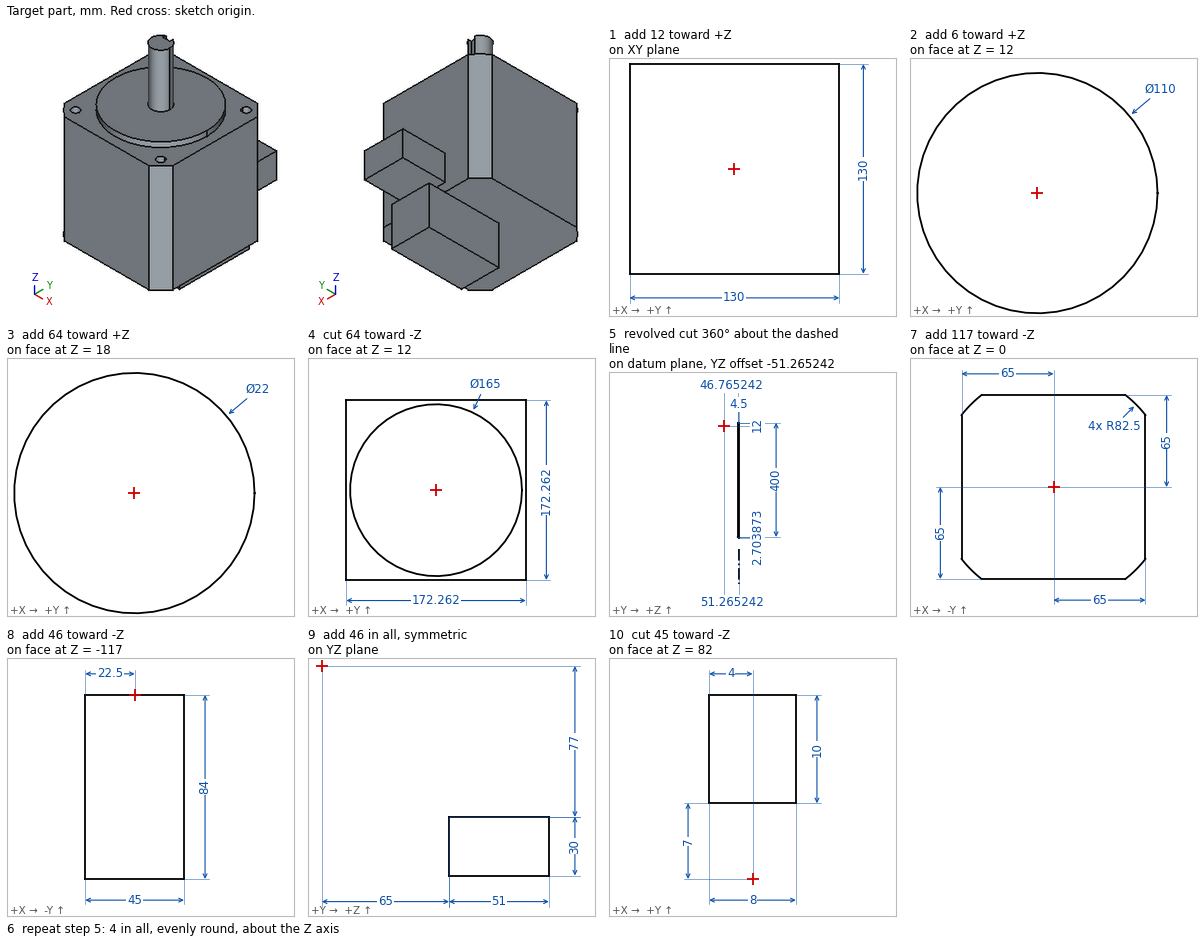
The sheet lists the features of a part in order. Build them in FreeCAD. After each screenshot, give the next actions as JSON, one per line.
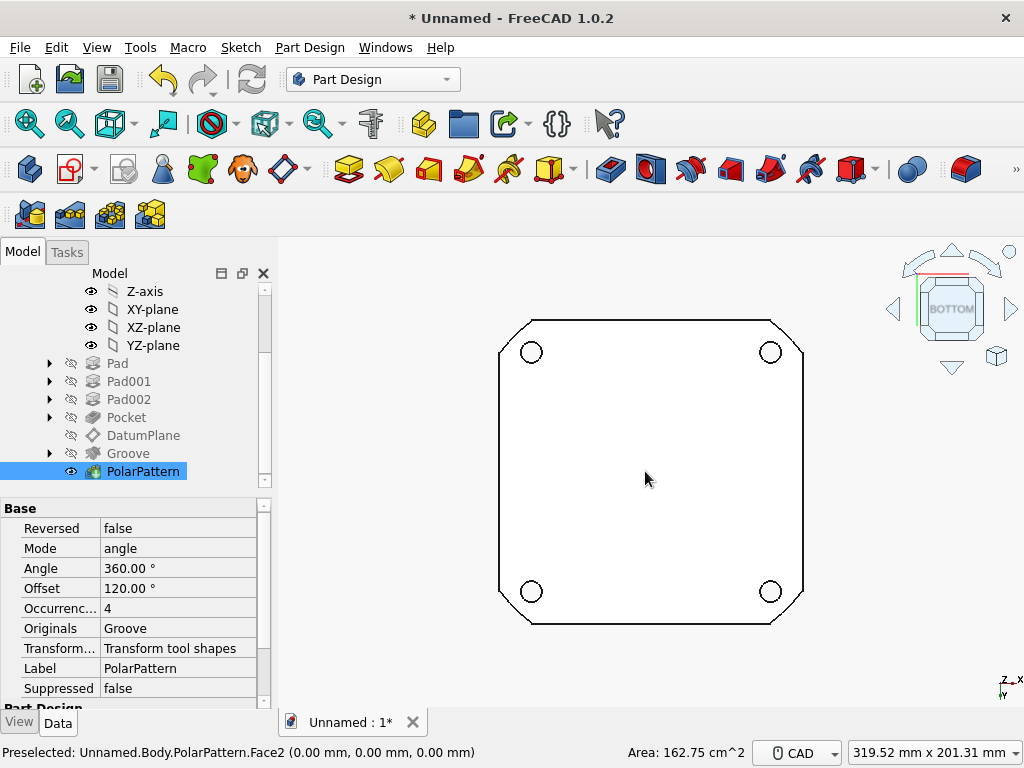
{"action": "left_click", "coordinate": [70, 170]}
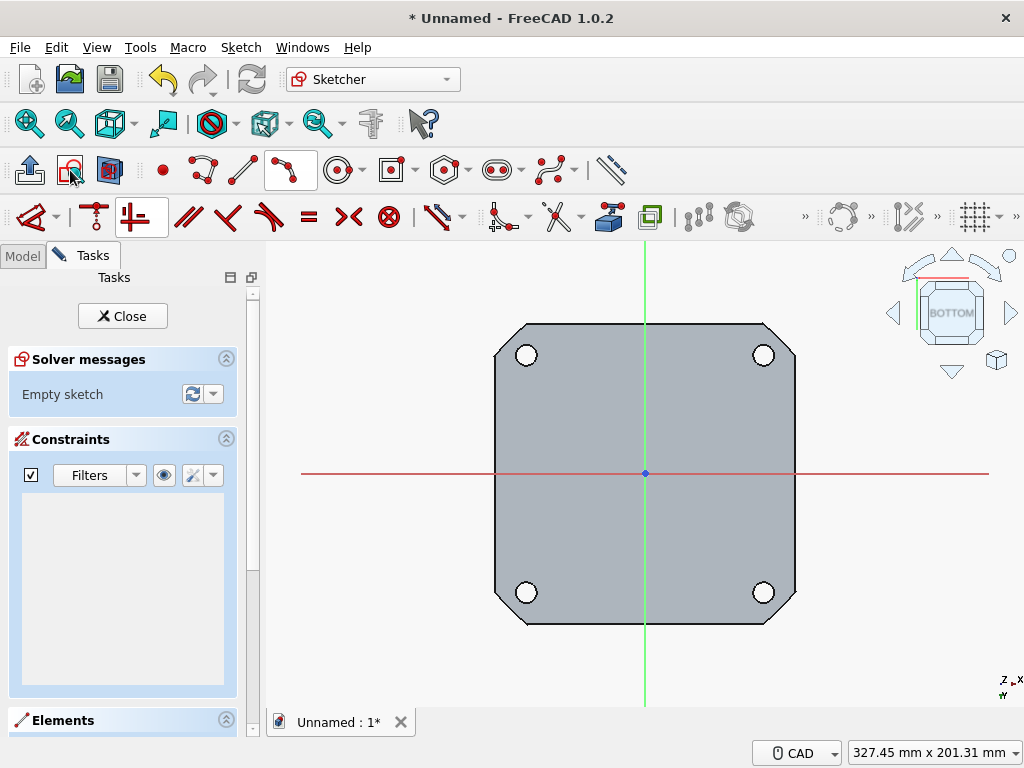
{"action": "key", "text": "g l"}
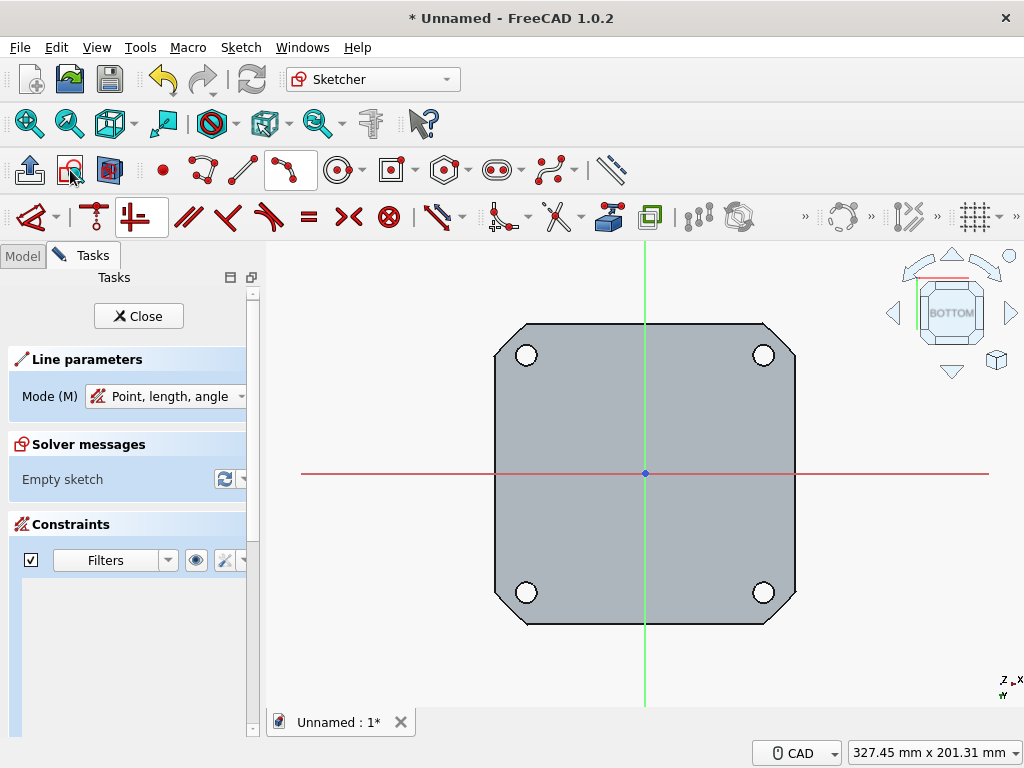
{"action": "left_click", "coordinate": [795, 592]}
{"action": "left_click", "coordinate": [795, 356]}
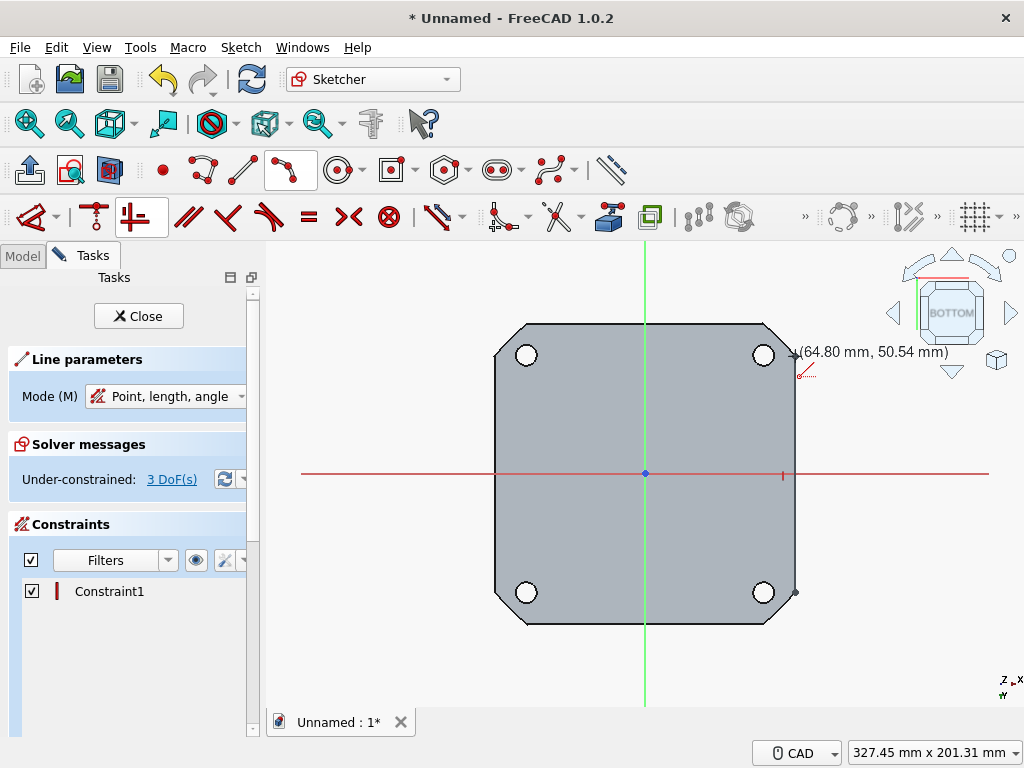
{"action": "left_click", "coordinate": [763, 324]}
{"action": "left_click", "coordinate": [527, 324]}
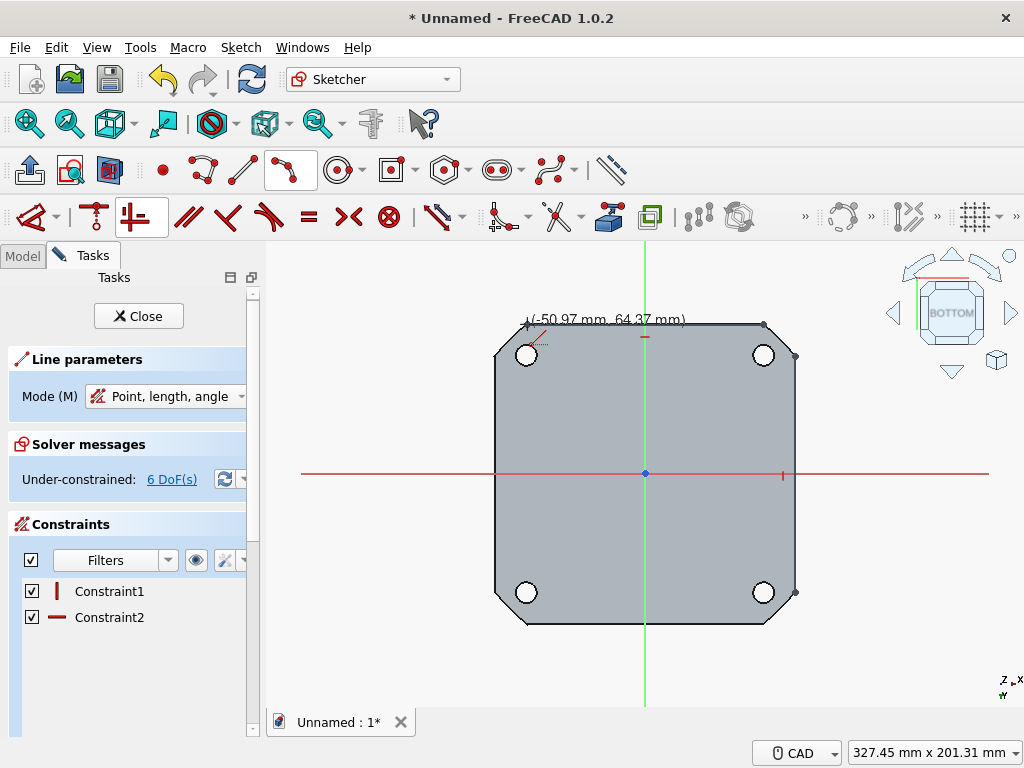
{"action": "left_click", "coordinate": [495, 356]}
{"action": "left_click", "coordinate": [495, 592]}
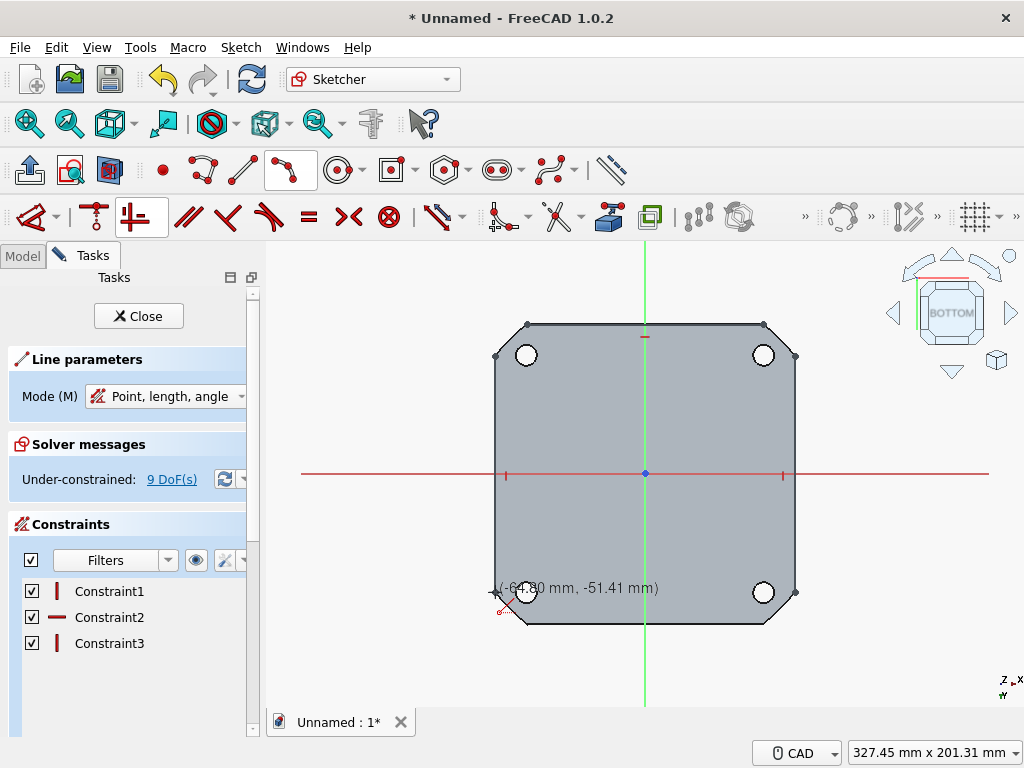
{"action": "left_click", "coordinate": [527, 624]}
{"action": "left_click", "coordinate": [763, 624]}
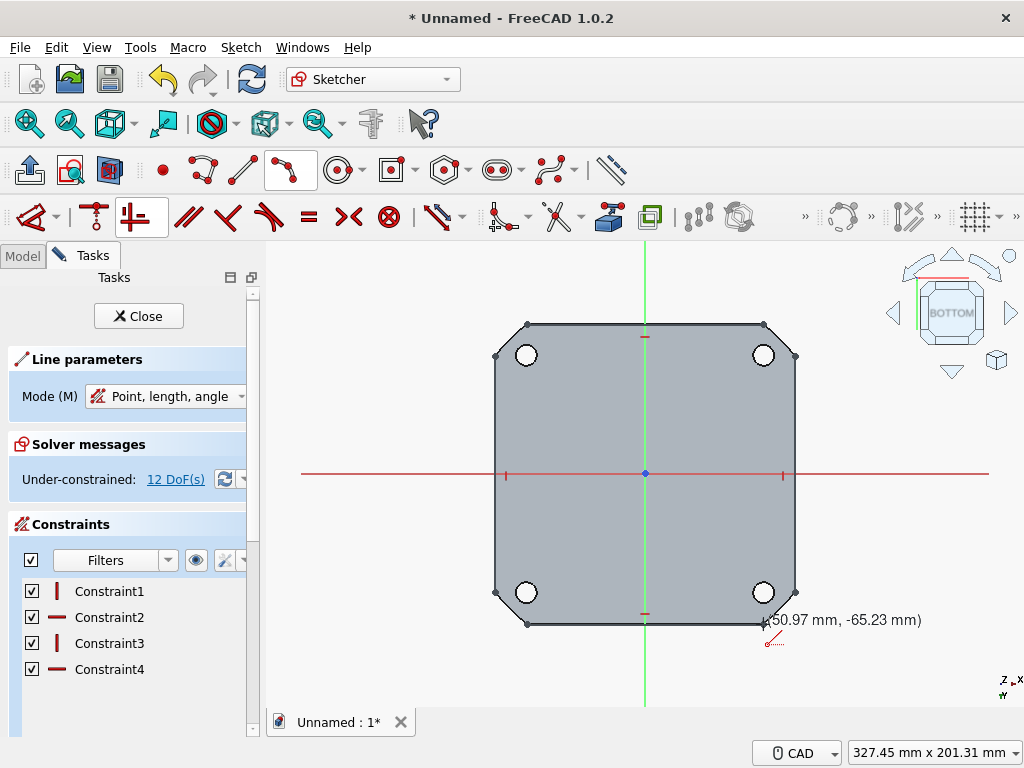
{"action": "left_click", "coordinate": [284, 170]}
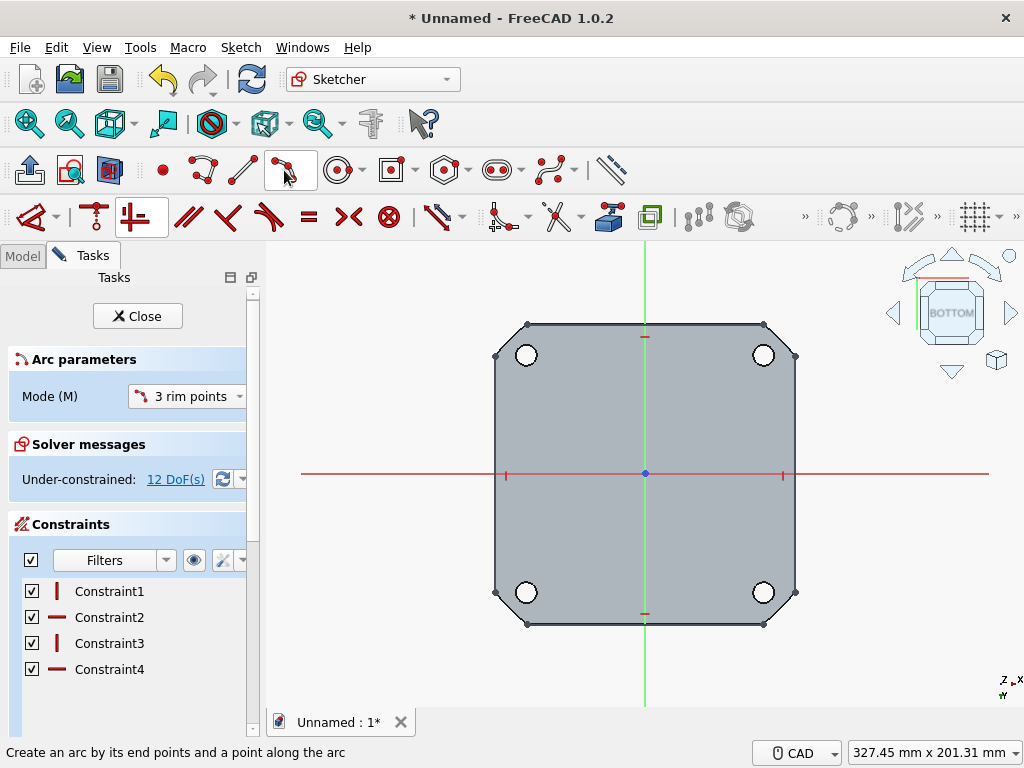
{"action": "left_click", "coordinate": [795, 357]}
{"action": "left_click", "coordinate": [763, 325]}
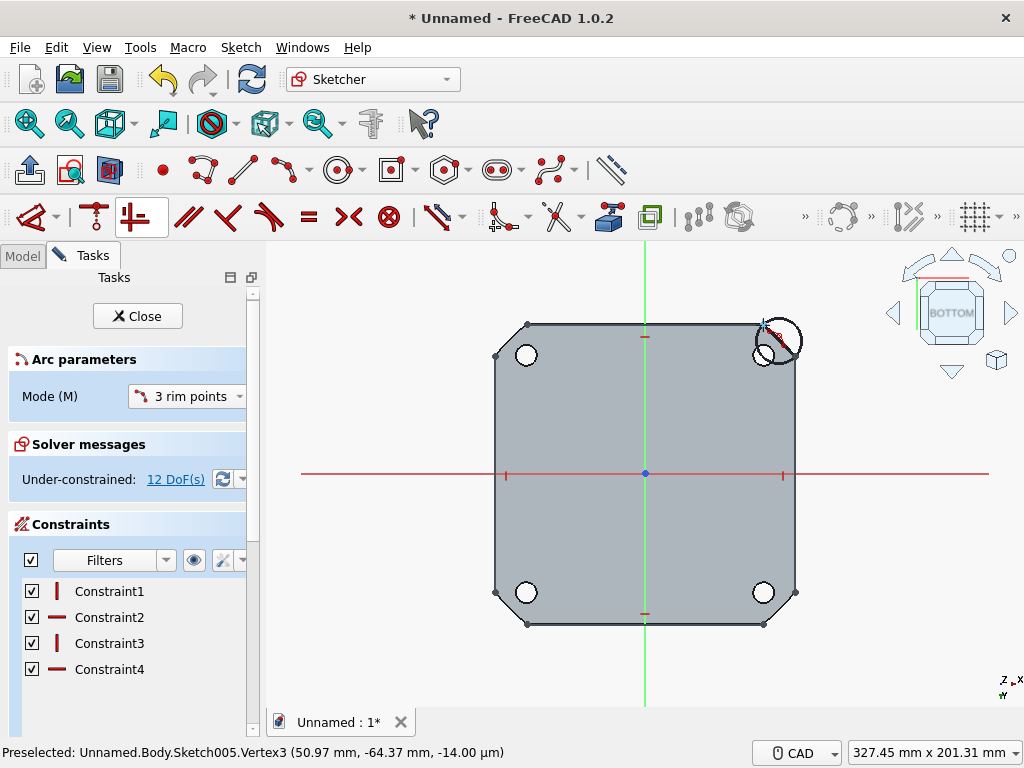
{"action": "scroll", "coordinate": [780, 339], "scroll_direction": "up", "scroll_amount": 13}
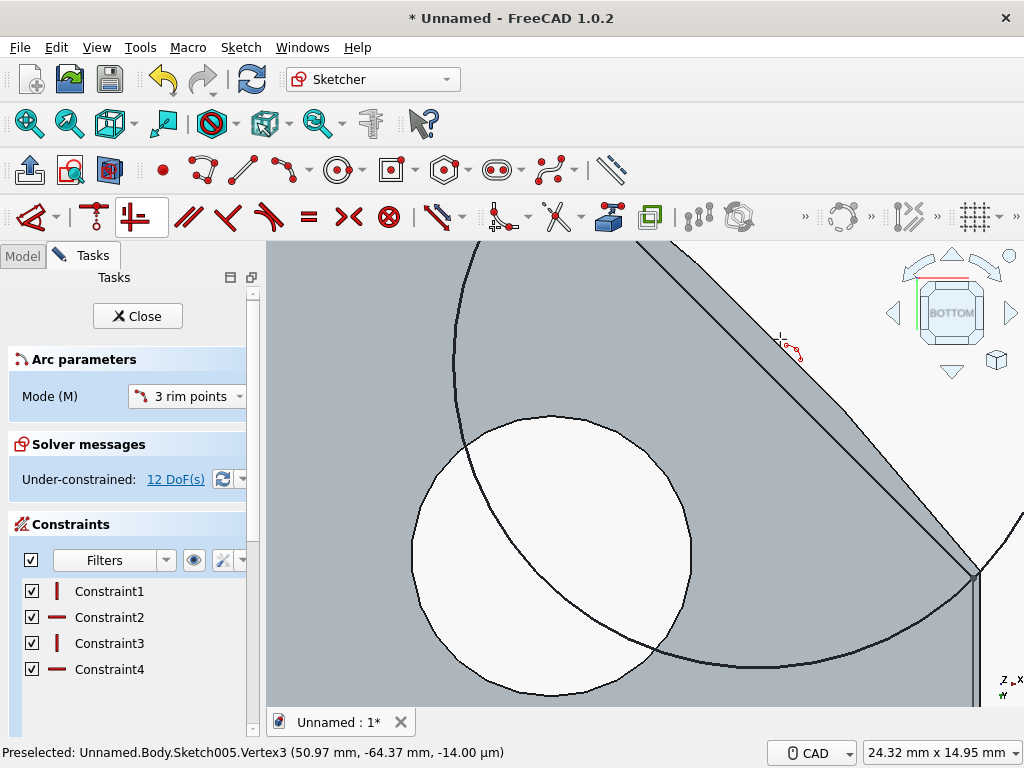
{"action": "left_click", "coordinate": [772, 336]}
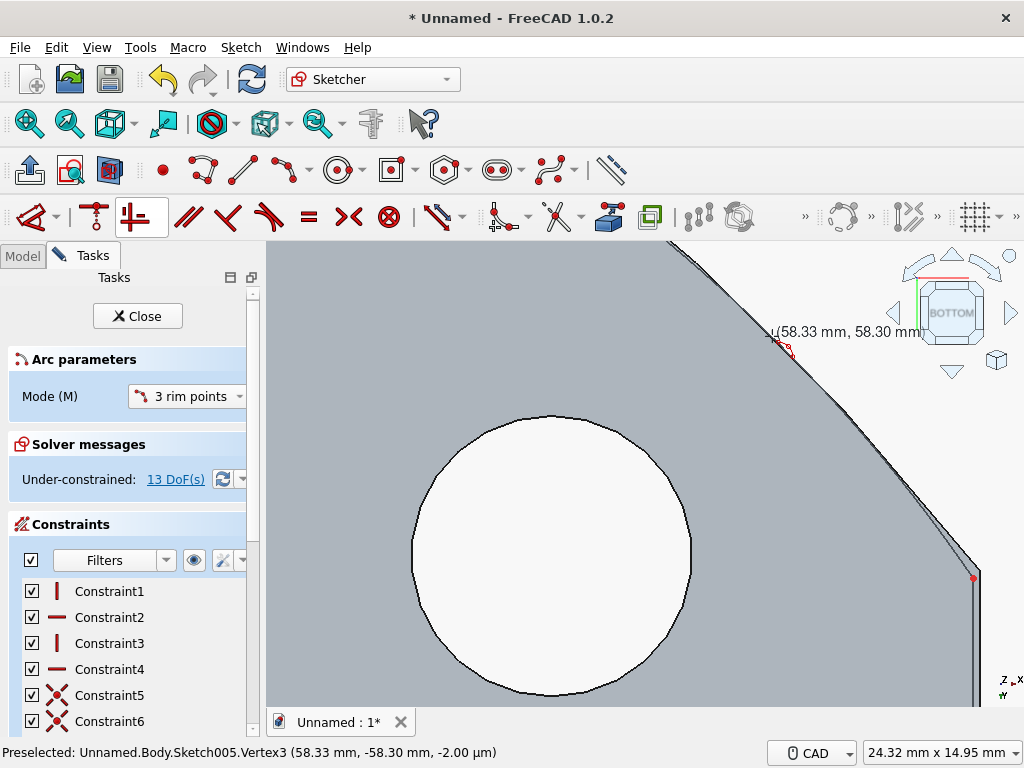
{"action": "scroll", "coordinate": [707, 339], "scroll_direction": "down", "scroll_amount": 13}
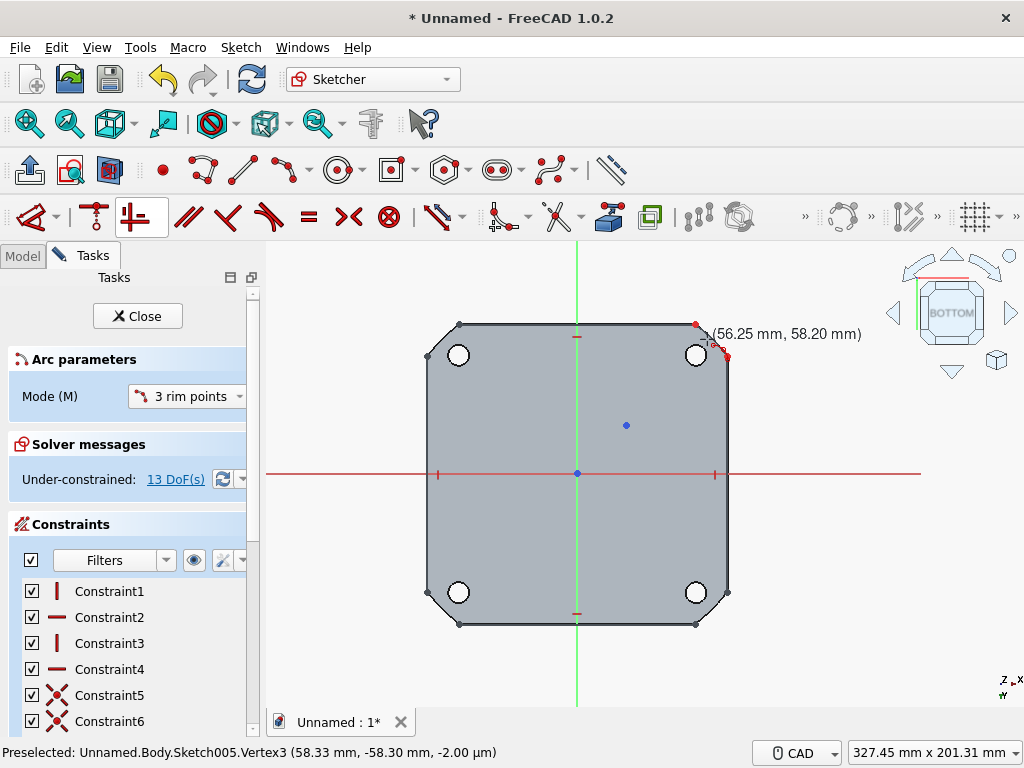
{"action": "left_click", "coordinate": [459, 325]}
{"action": "left_click", "coordinate": [427, 357]}